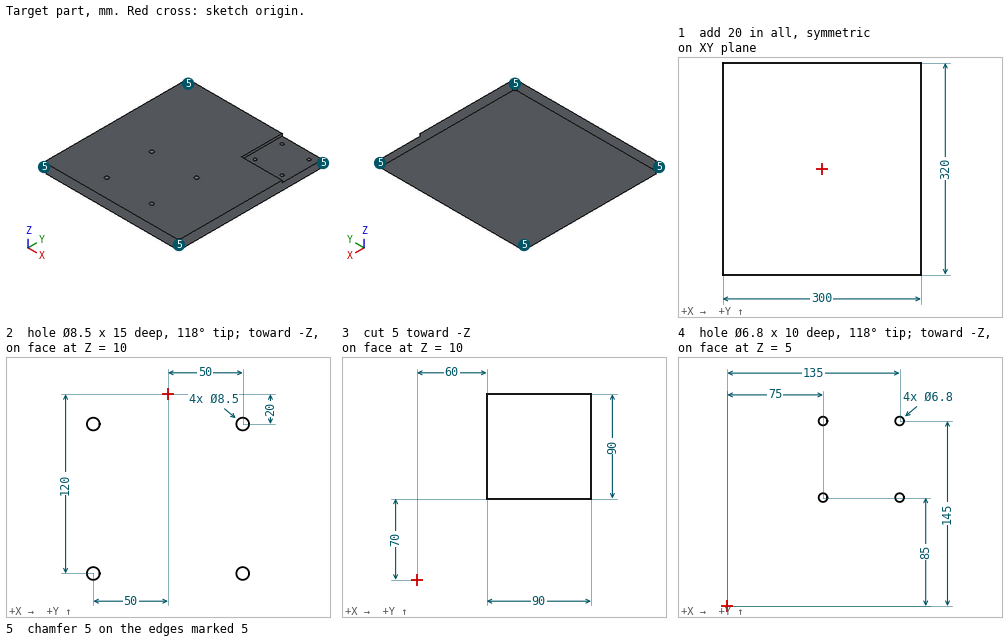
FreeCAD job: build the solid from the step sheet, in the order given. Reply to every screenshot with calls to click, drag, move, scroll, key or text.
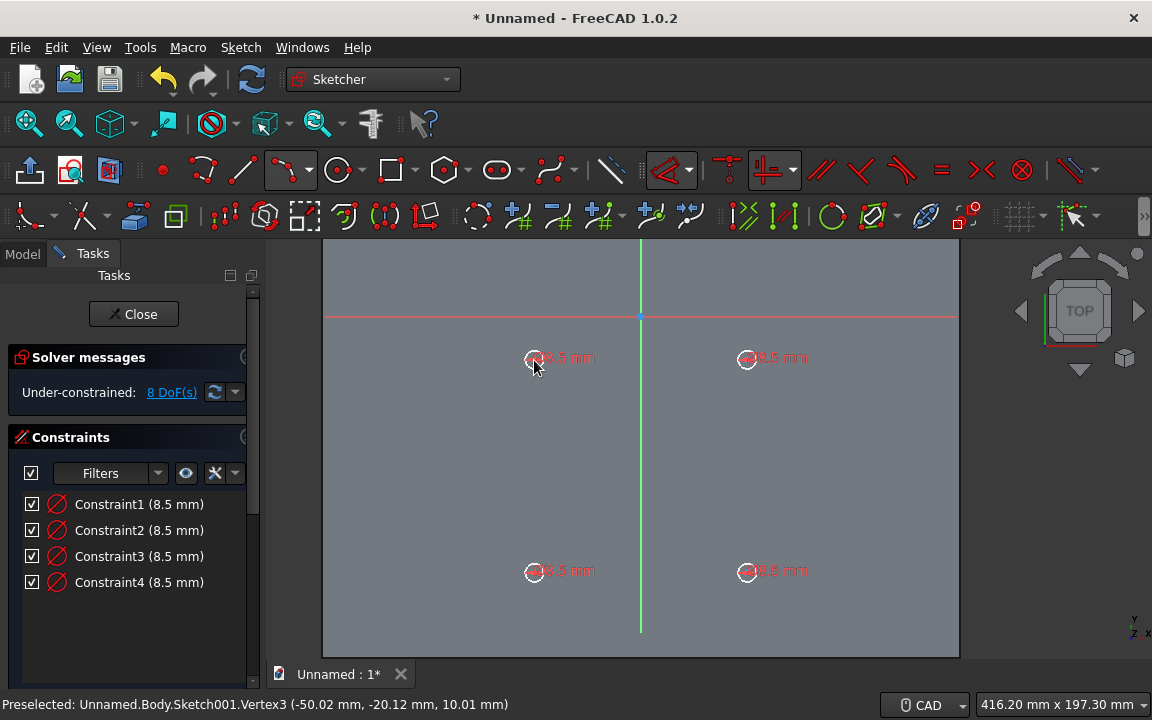
key(v)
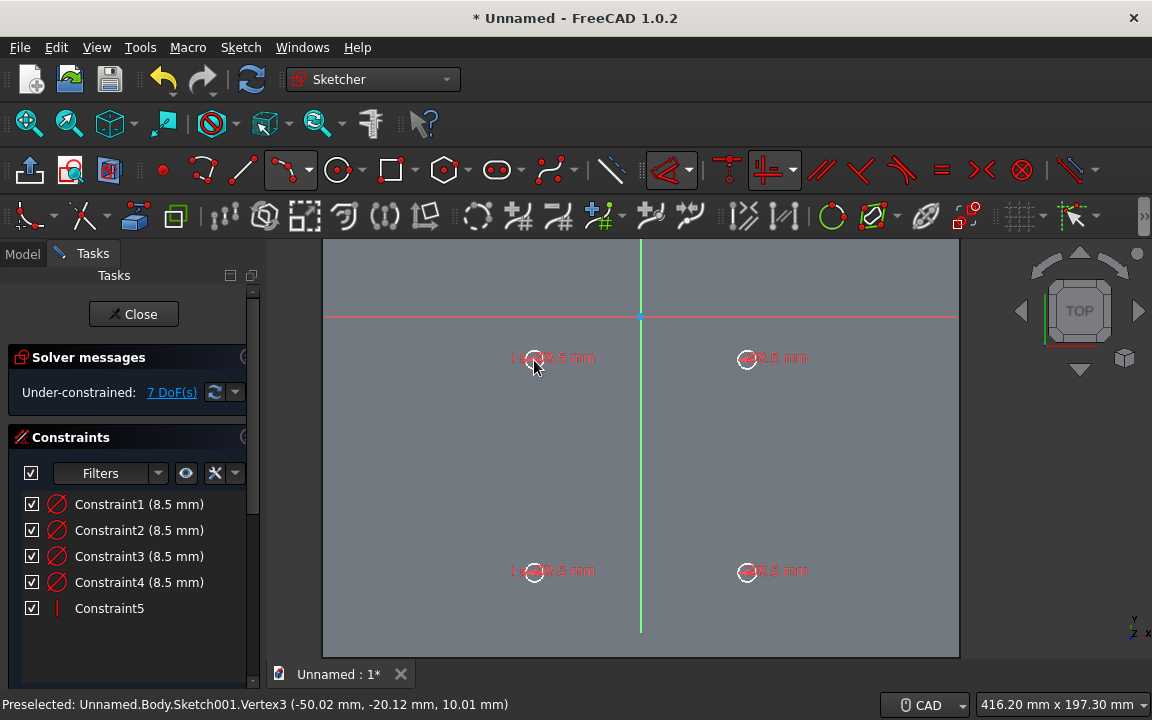
click(747, 360)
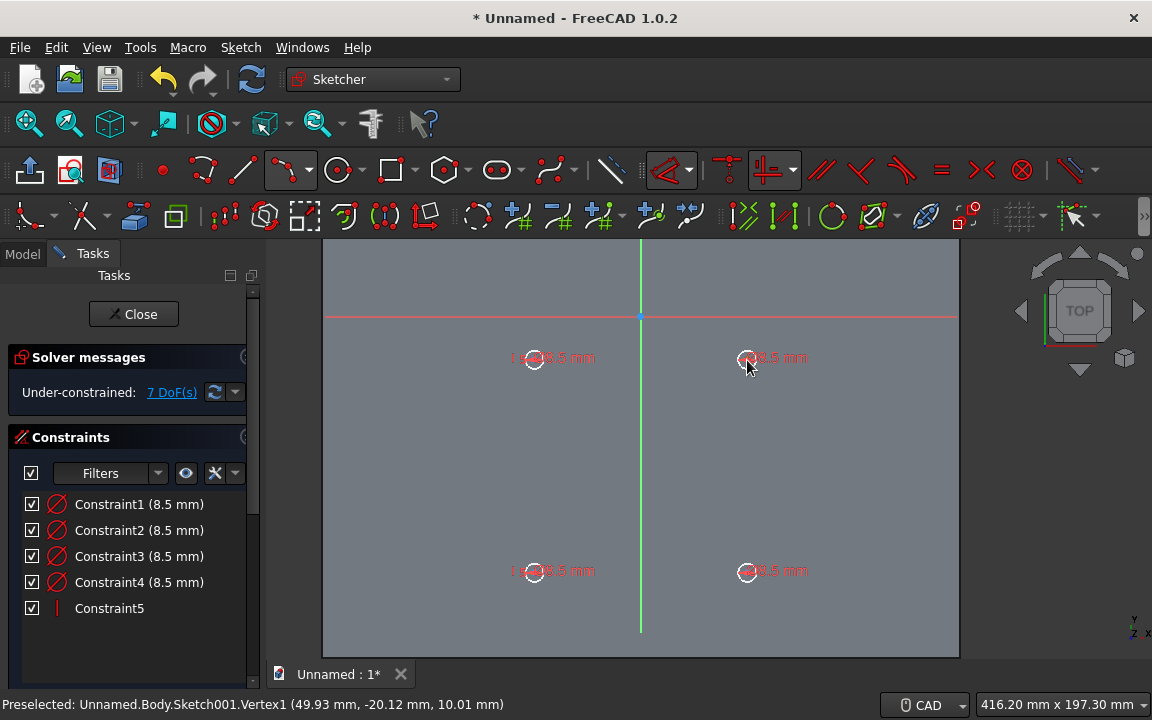
click(534, 360)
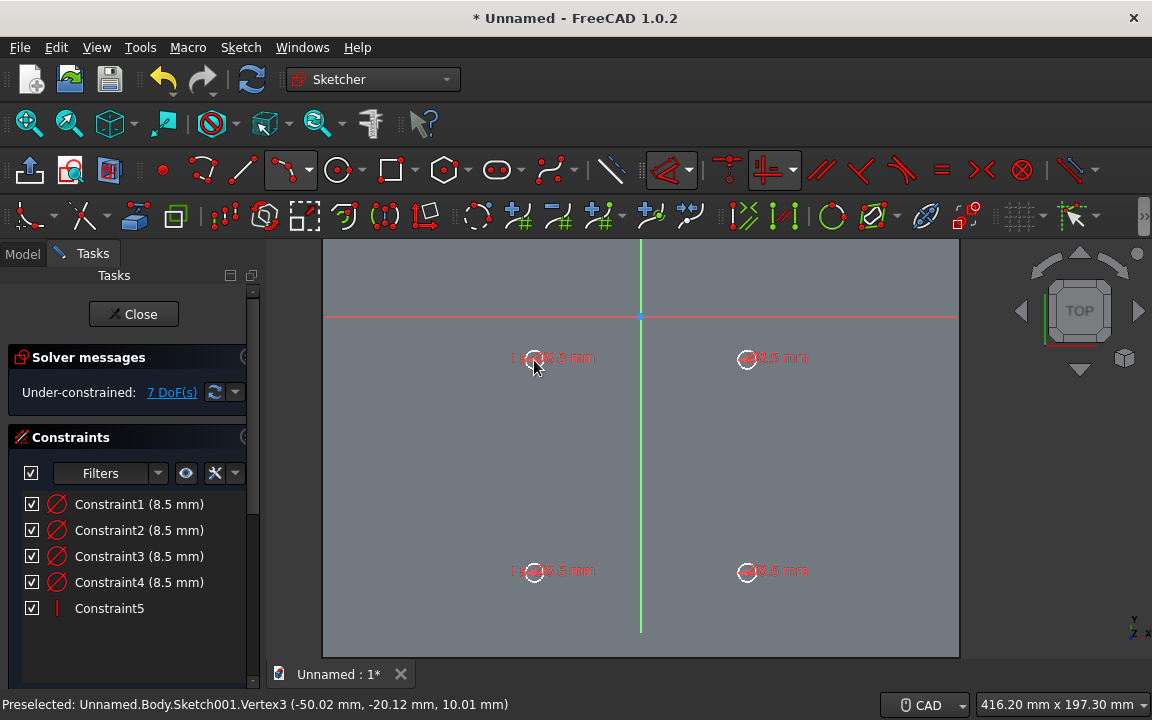
key(h)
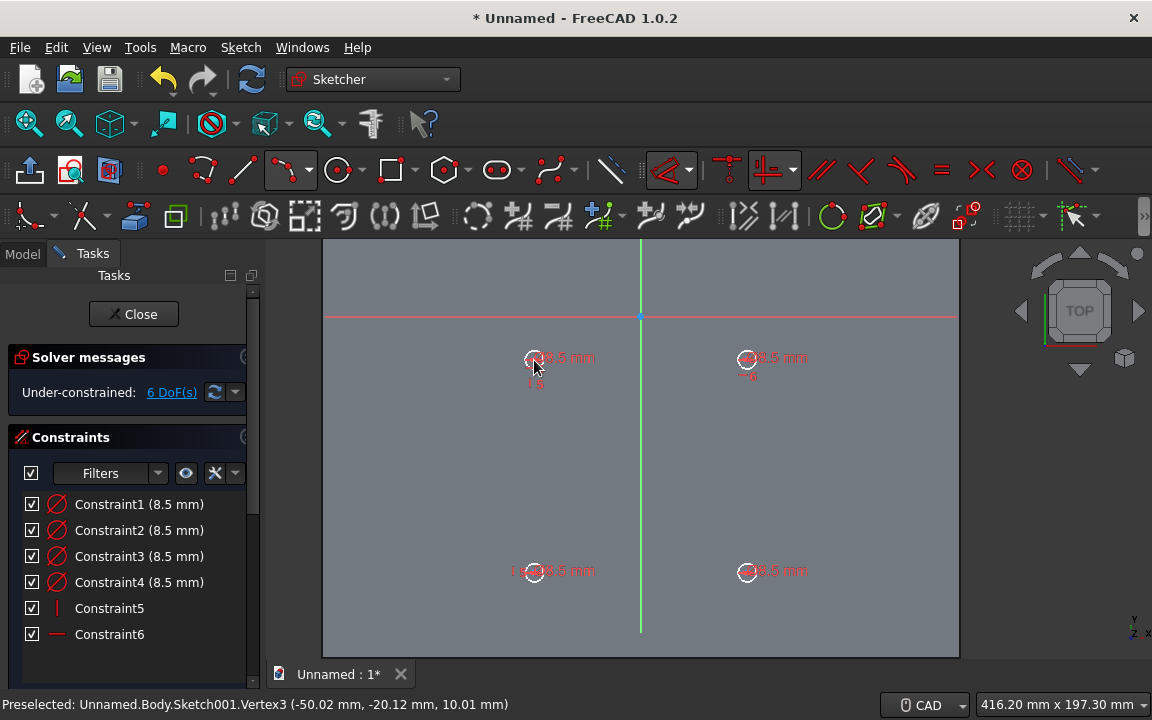
click(747, 360)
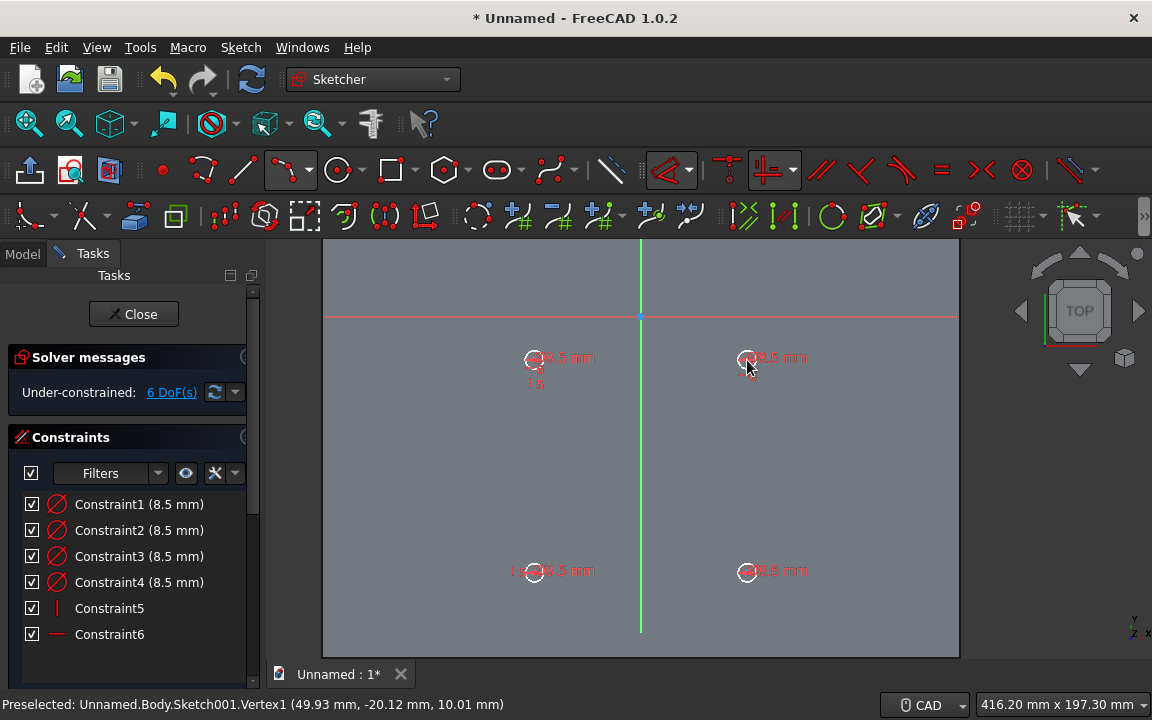
click(747, 573)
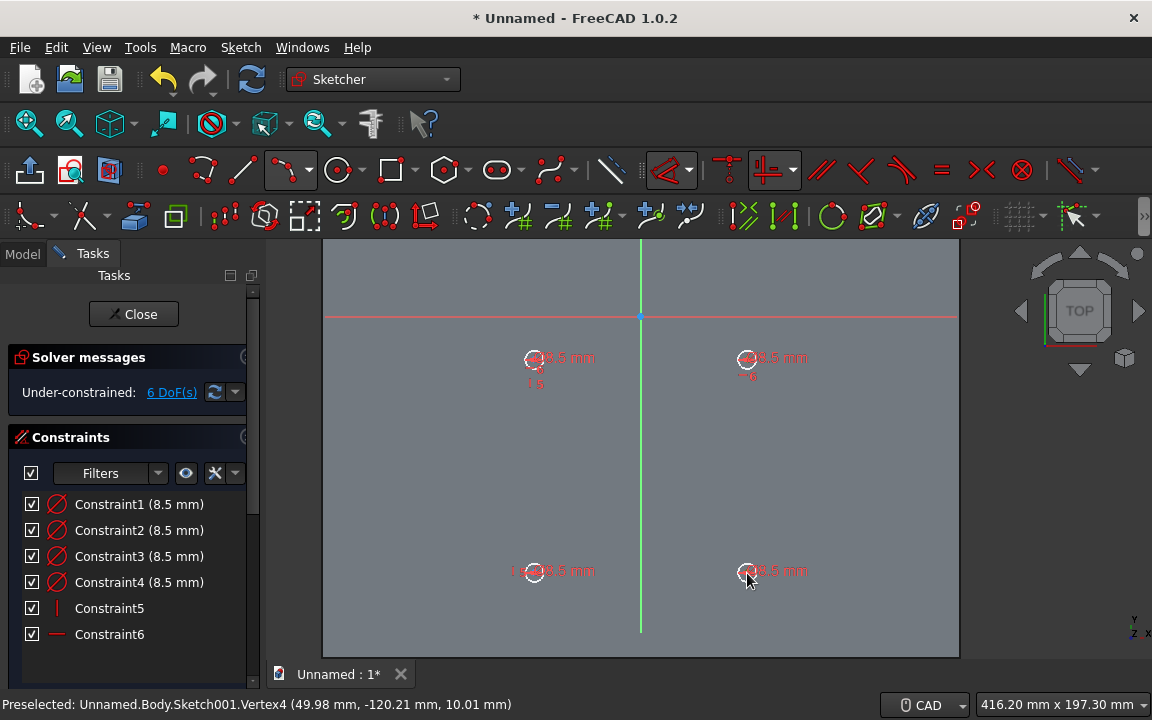
key(v)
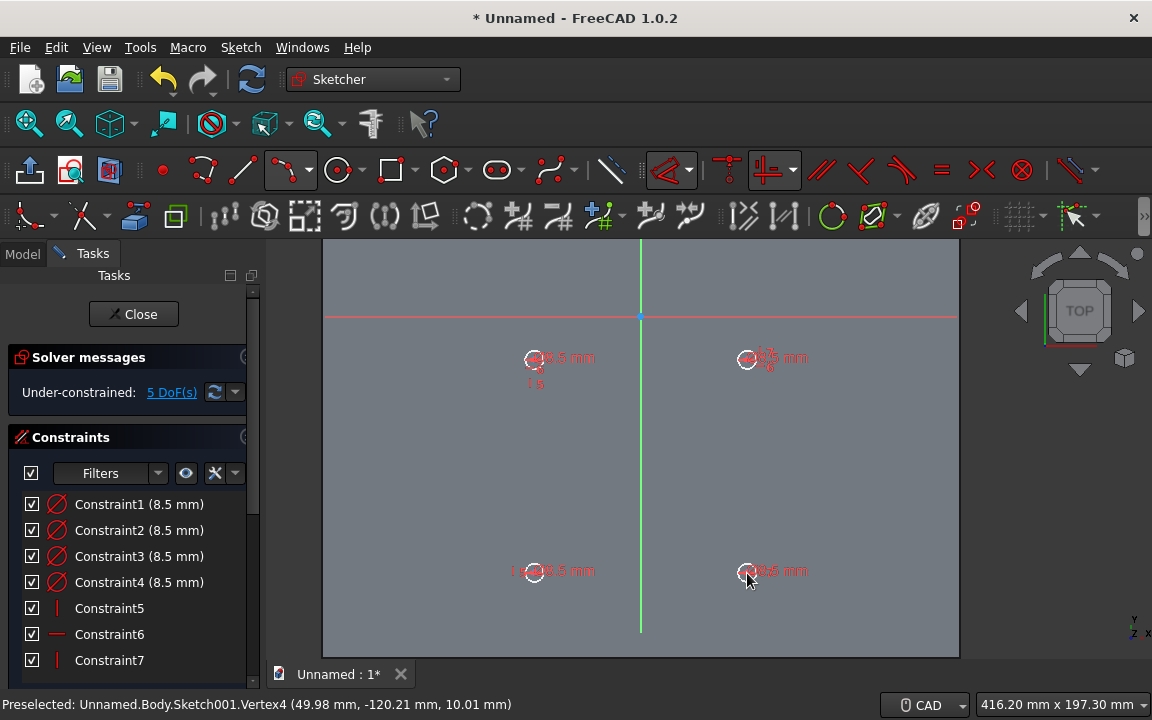
click(534, 573)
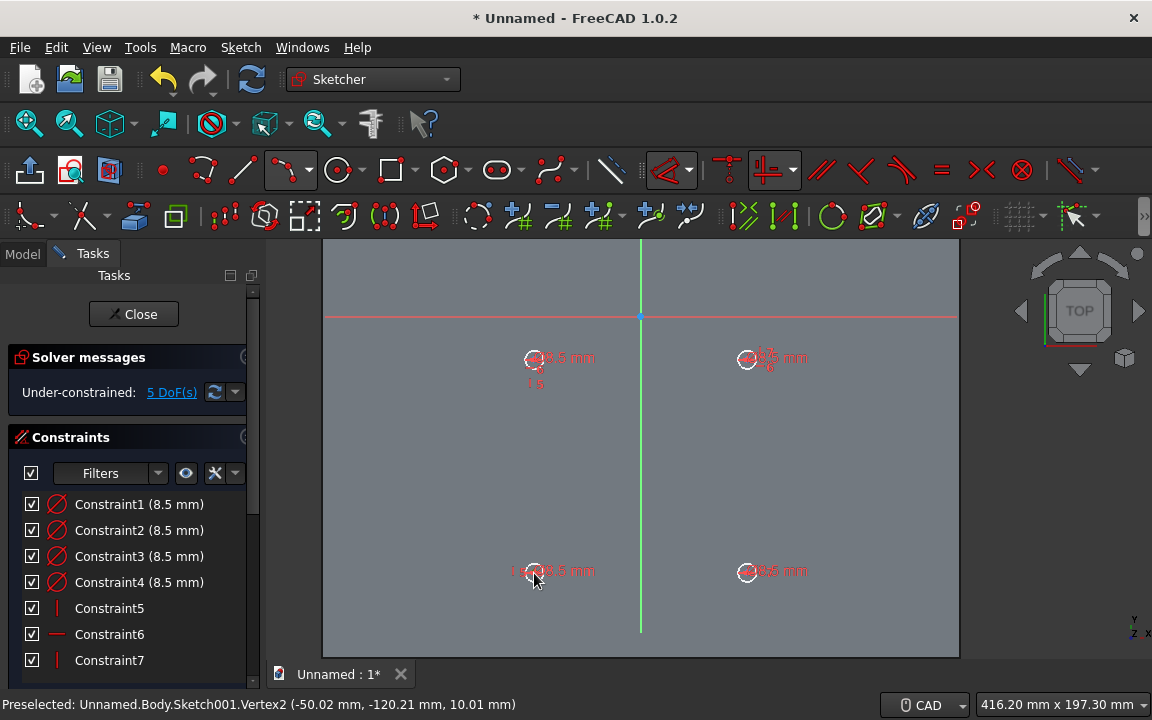
click(747, 573)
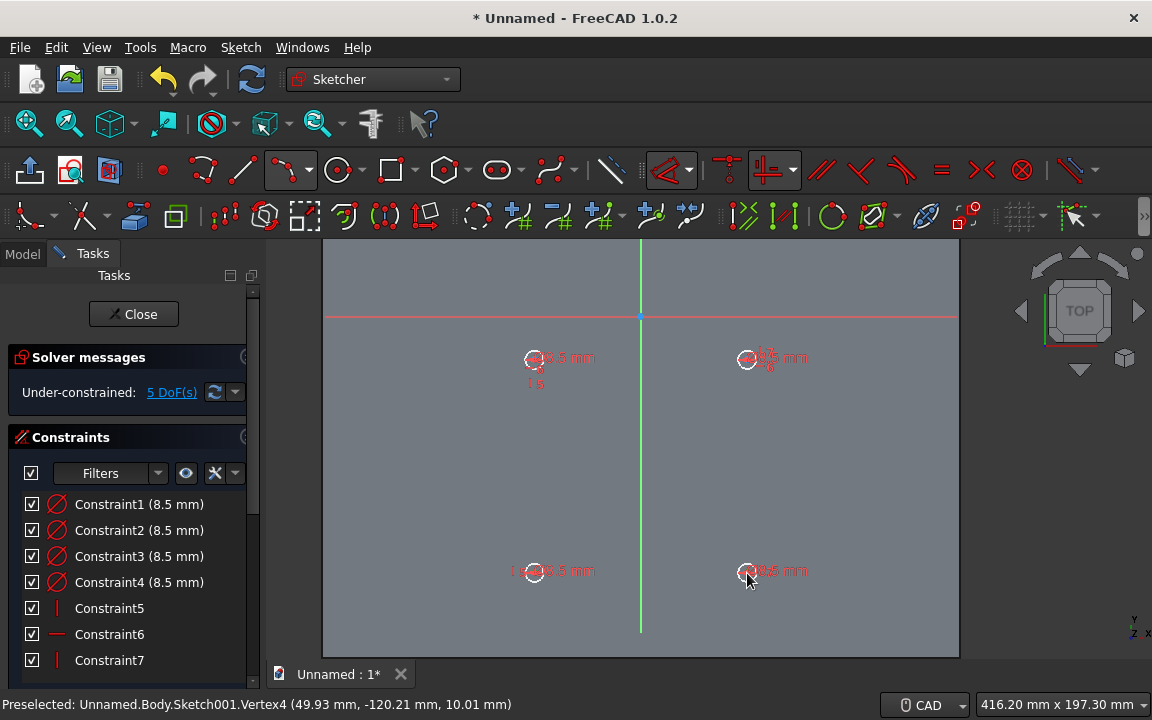
key(h)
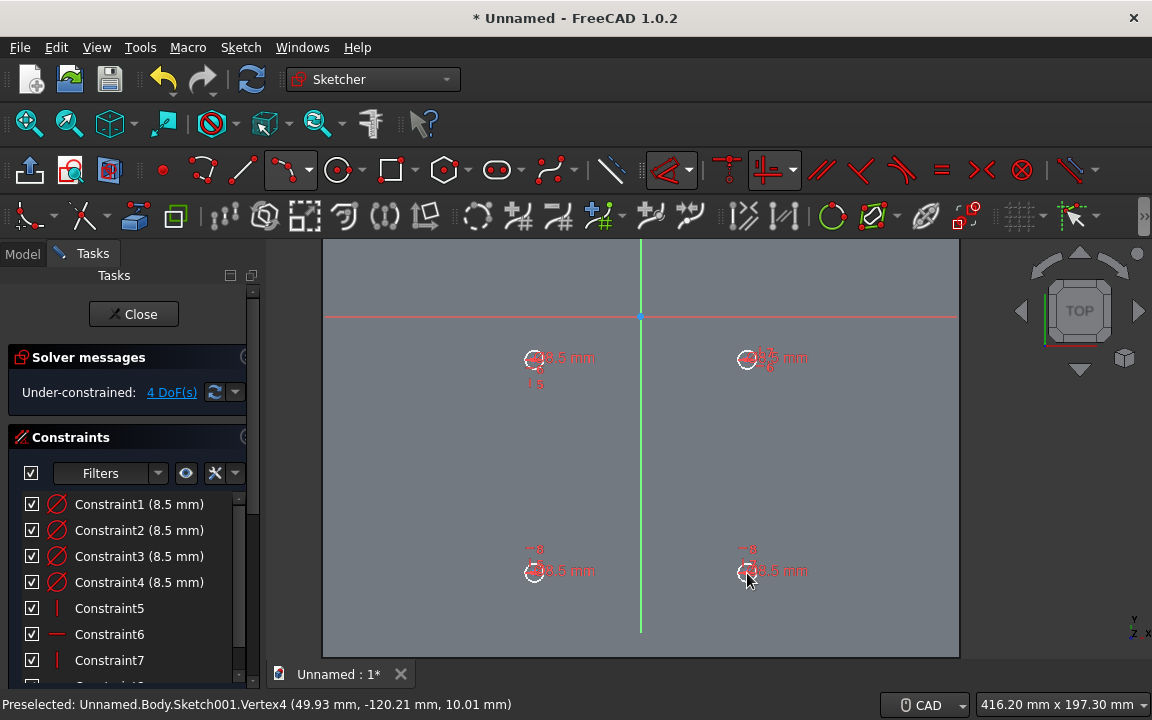
click(747, 360)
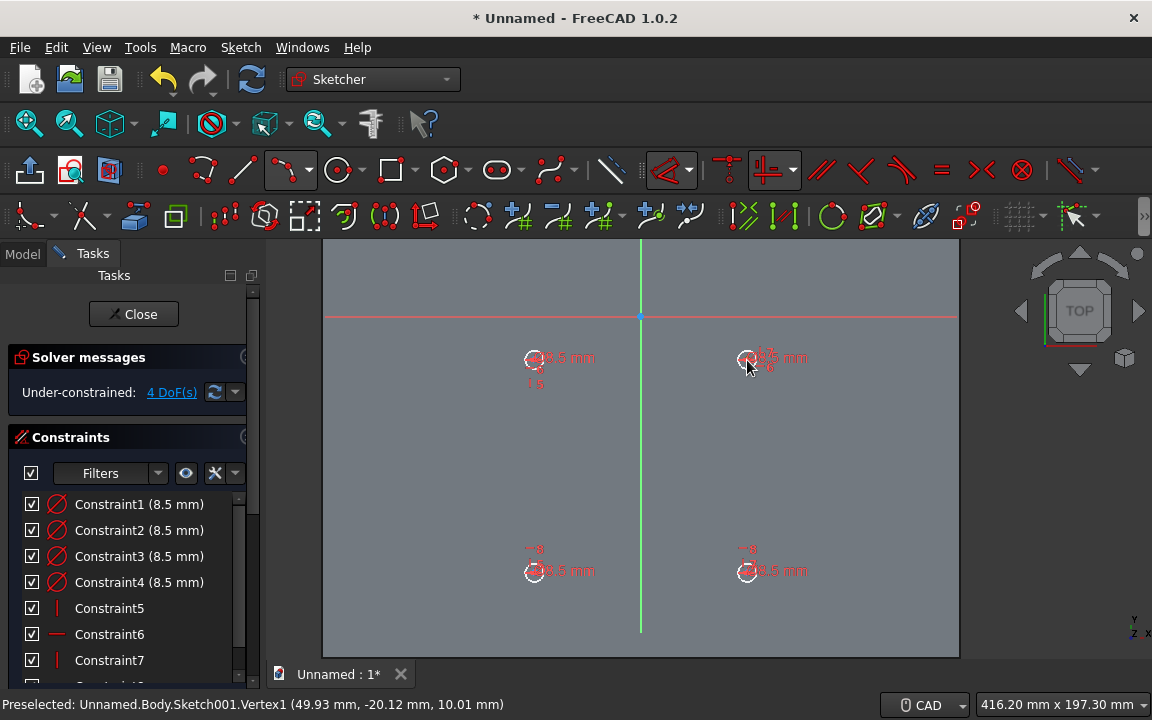
key(l)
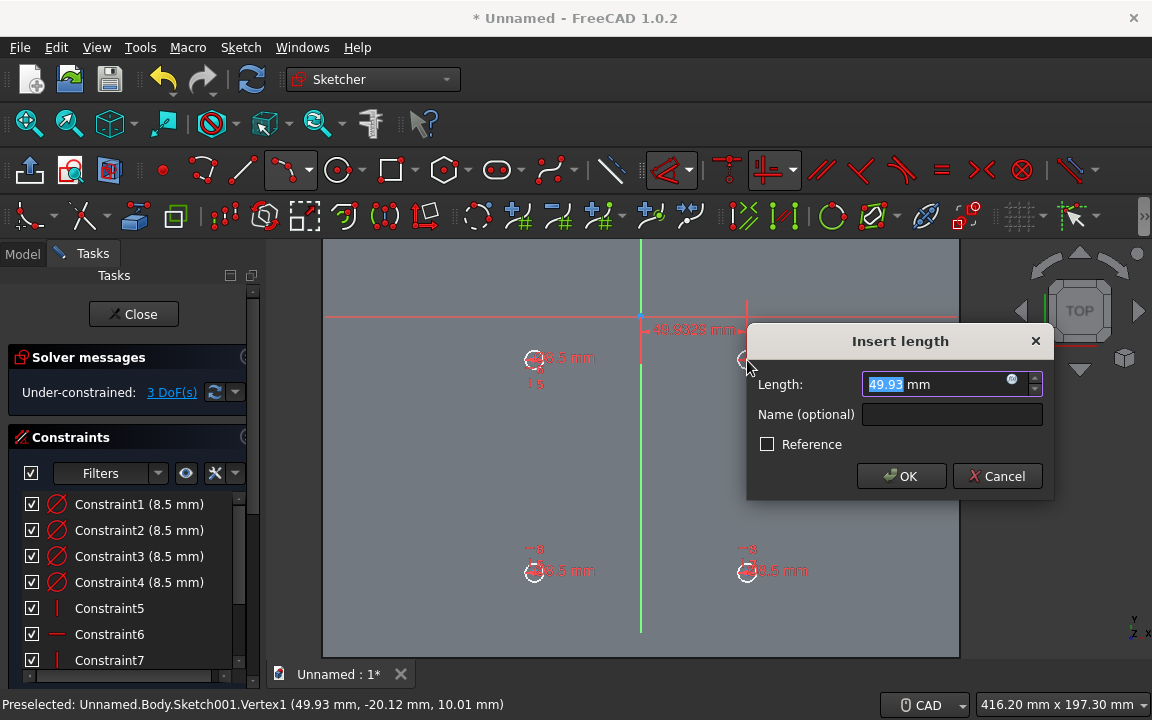
text(50)
key(Return)